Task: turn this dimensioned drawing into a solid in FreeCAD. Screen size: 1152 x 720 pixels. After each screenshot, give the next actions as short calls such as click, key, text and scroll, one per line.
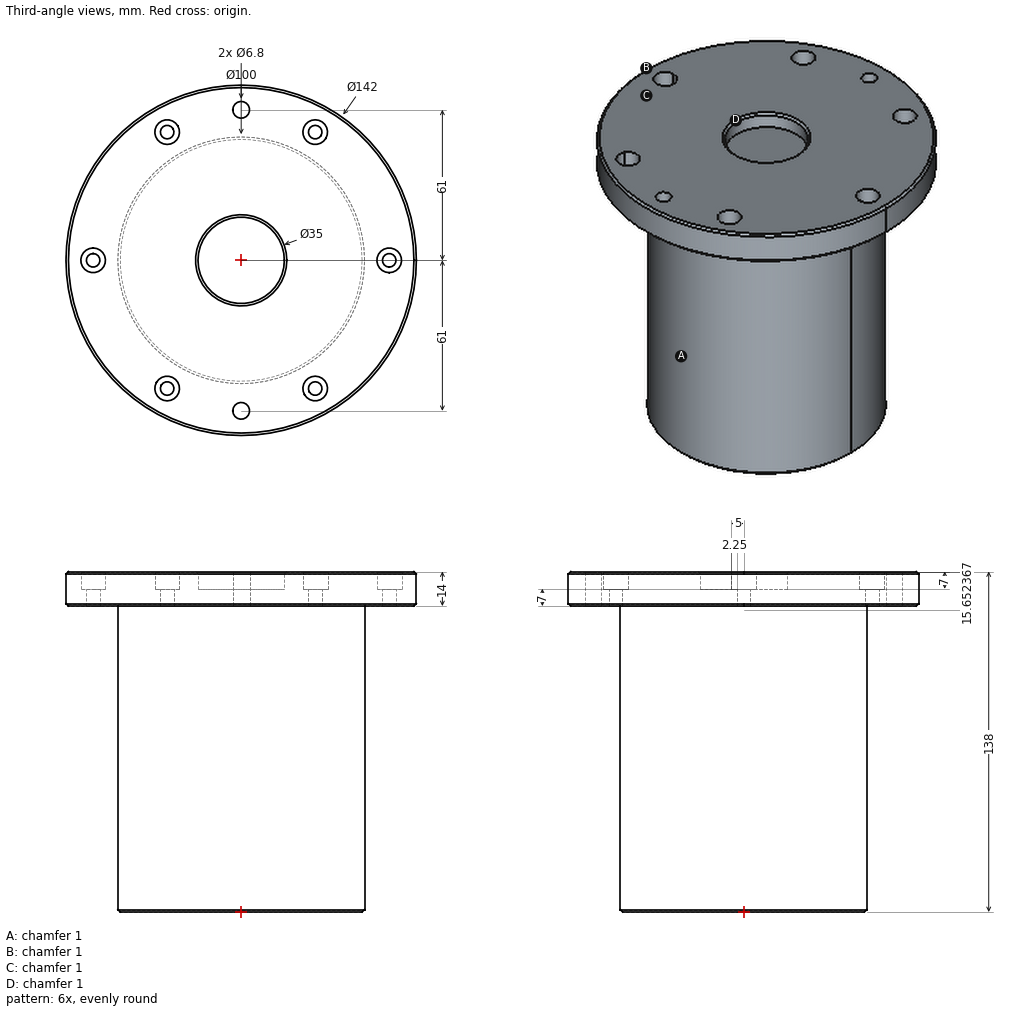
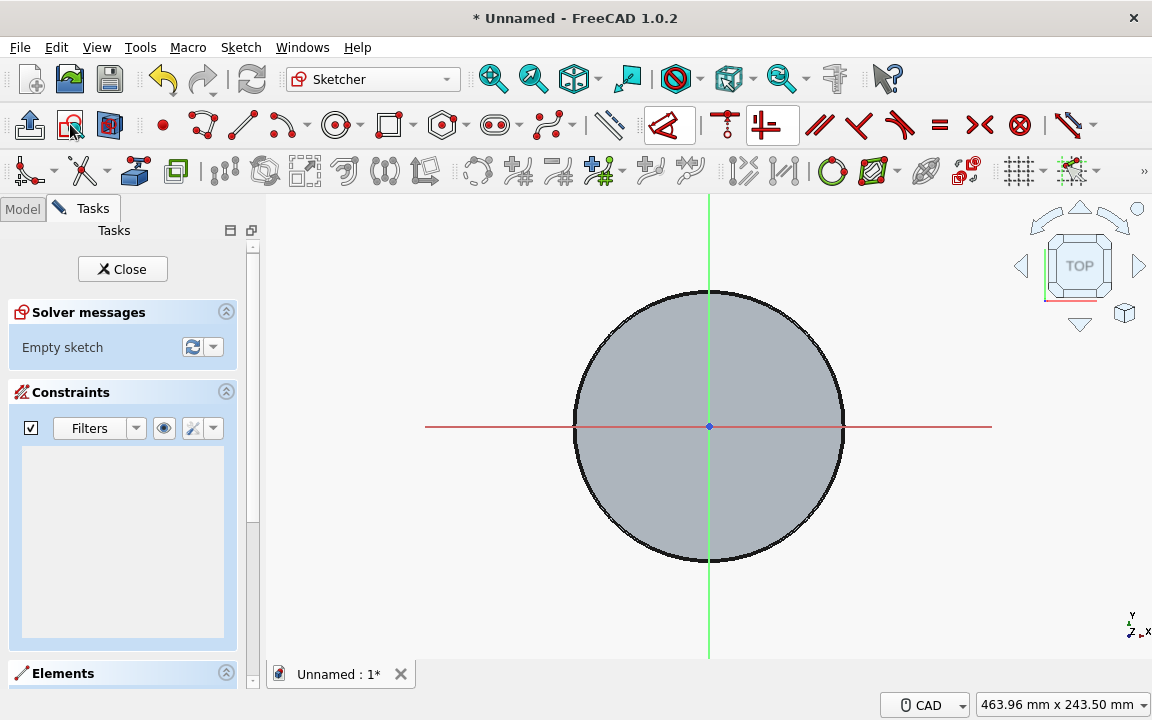
scroll(731, 426, up, 7)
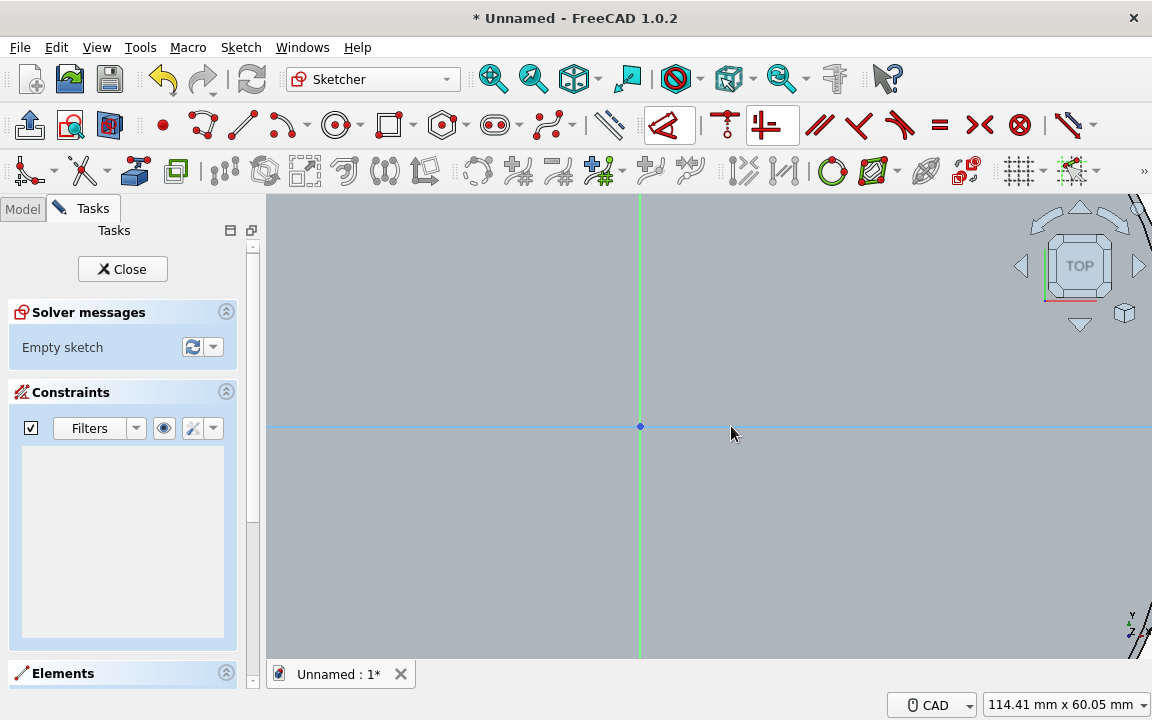
click(336, 126)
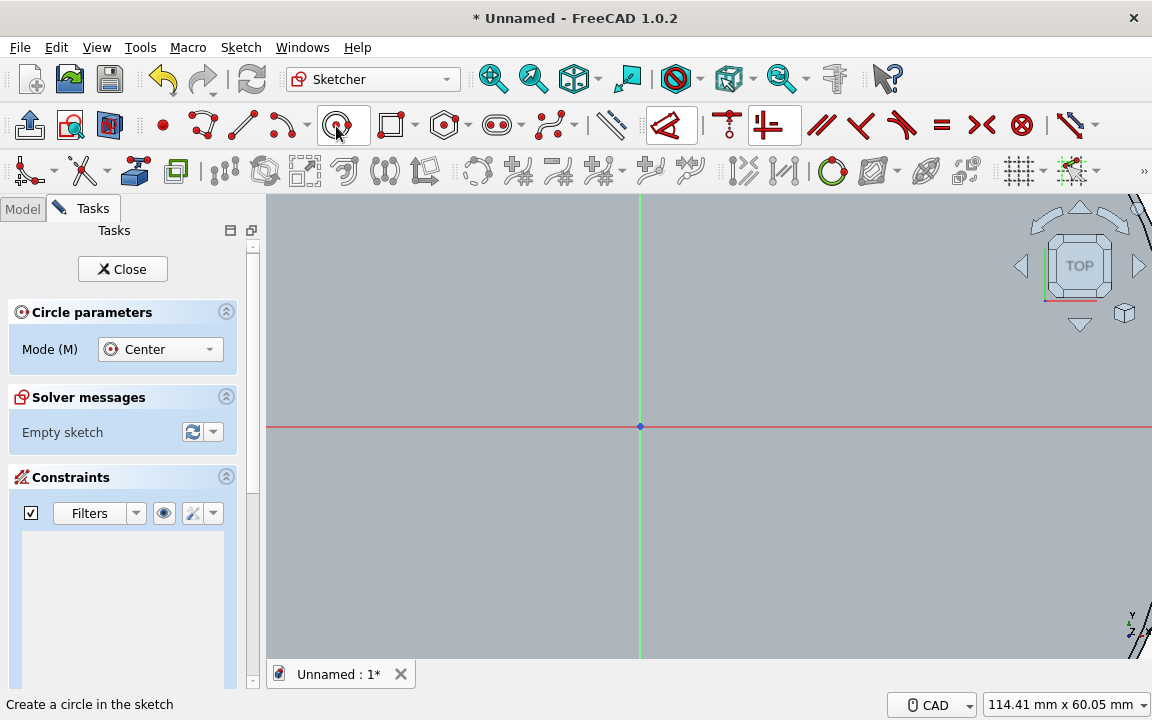
click(640, 426)
click(736, 331)
key(Escape)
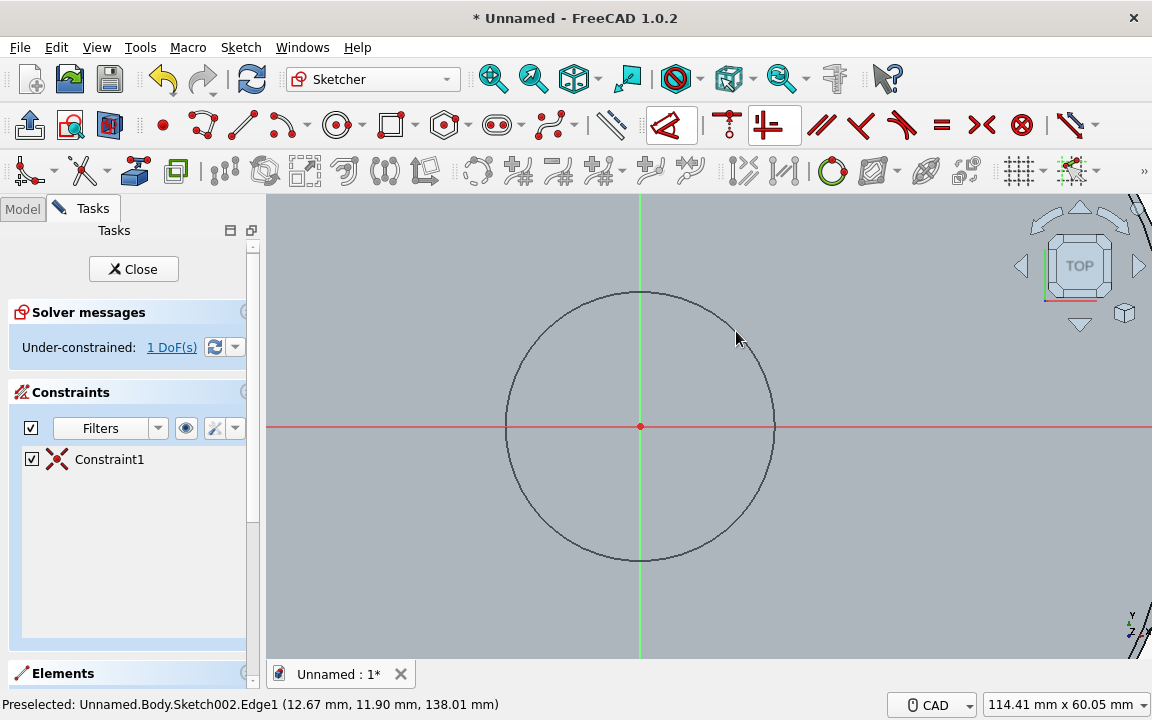
click(735, 331)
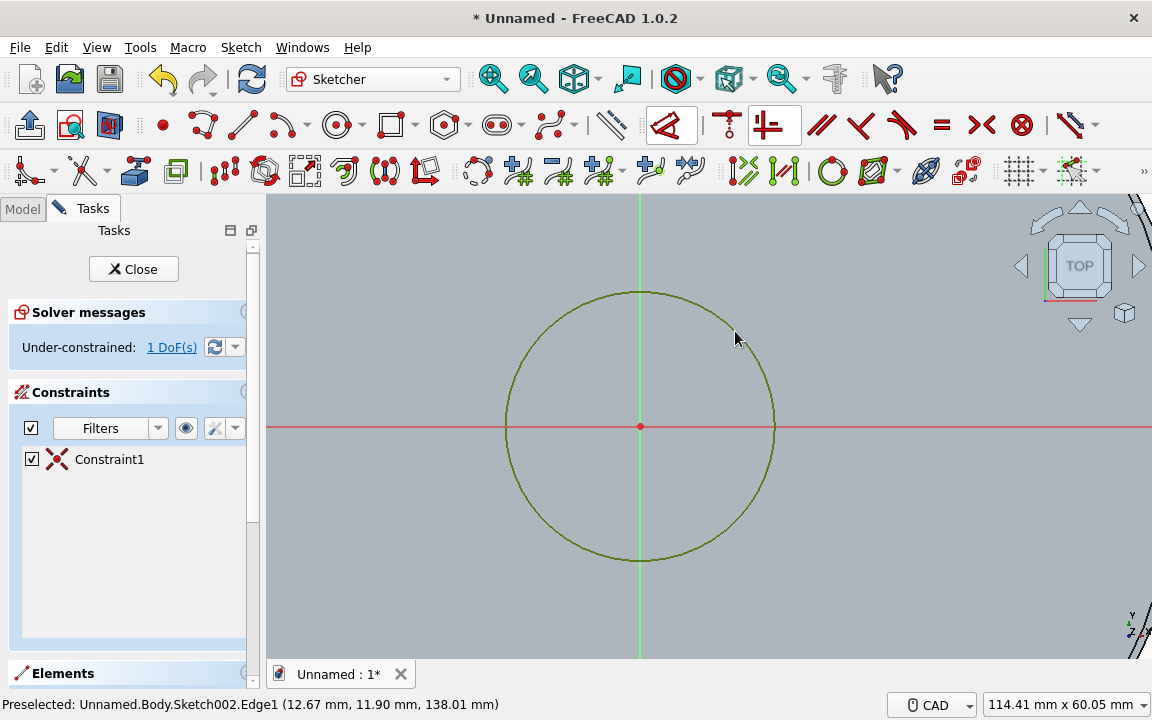
click(692, 126)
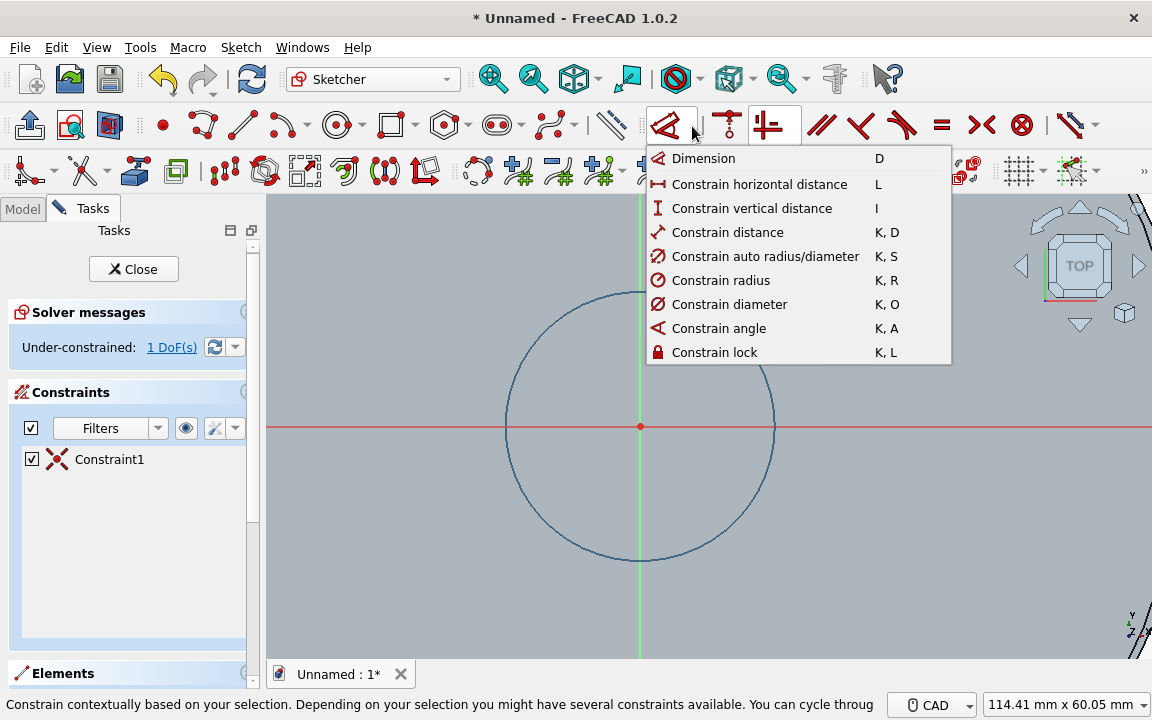
click(799, 304)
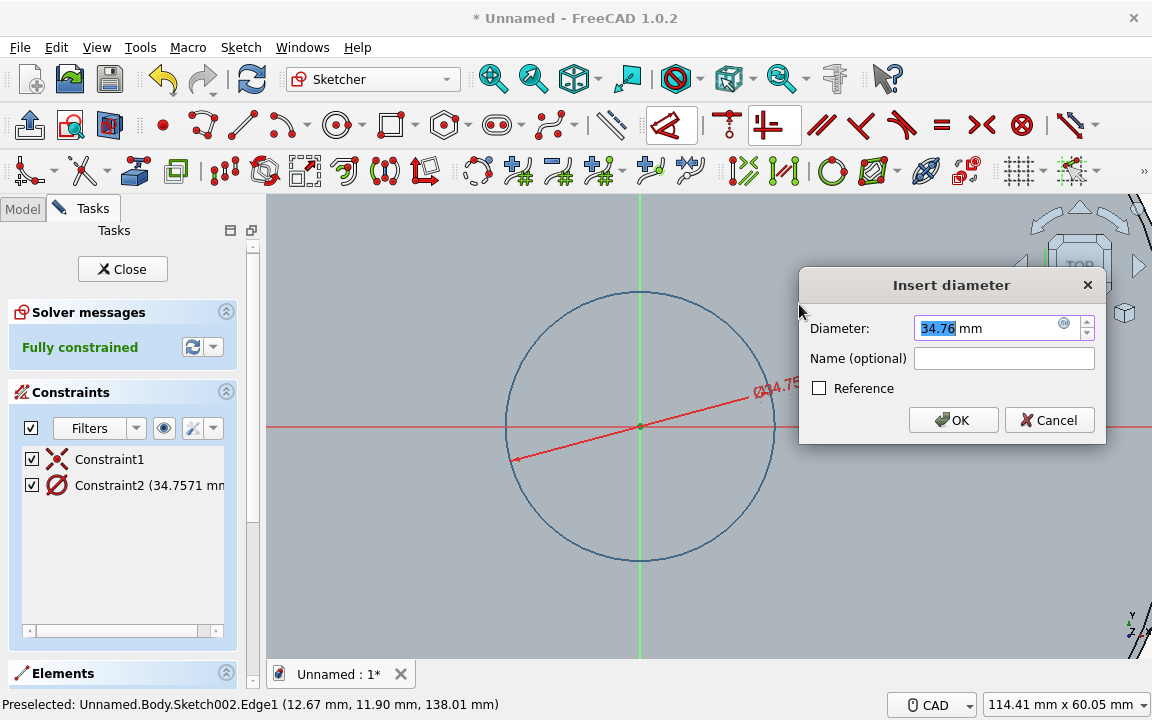
text(35)
key(Return)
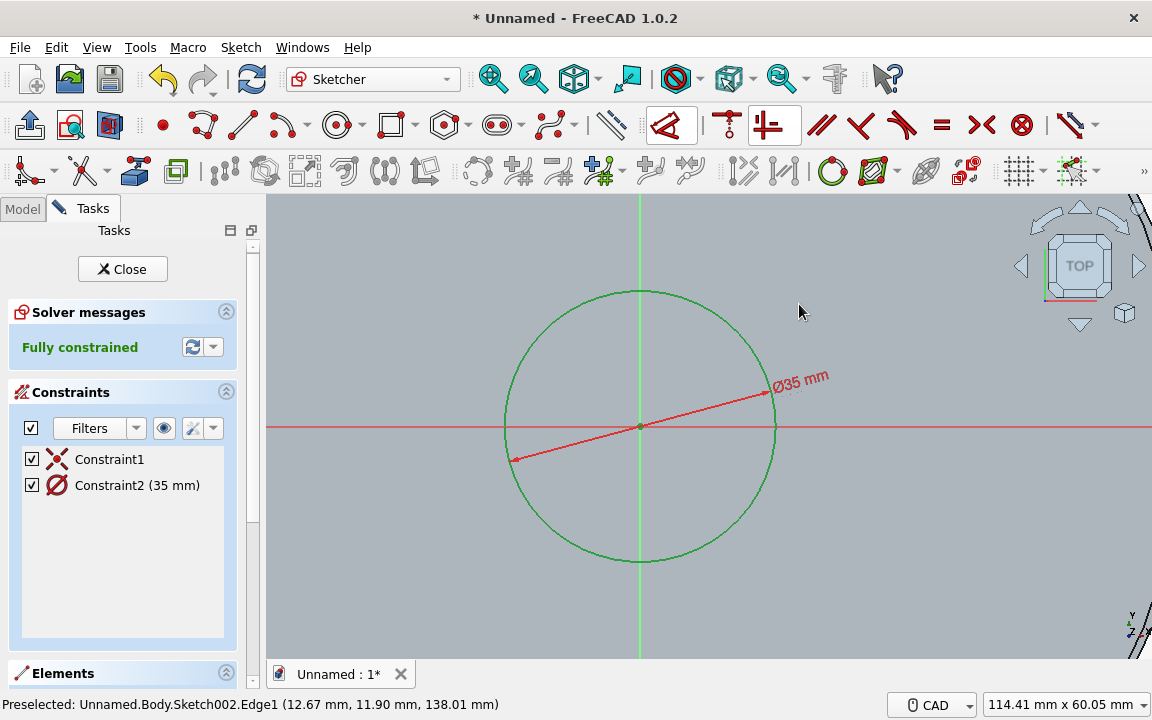
click(123, 269)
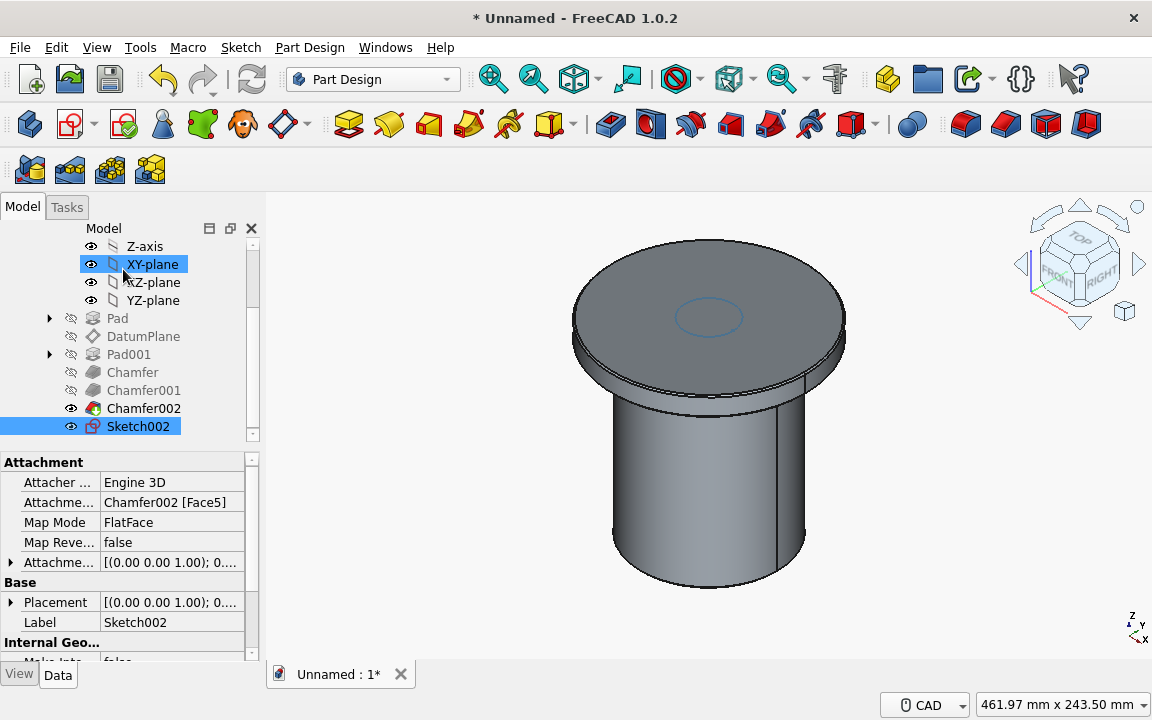
click(612, 124)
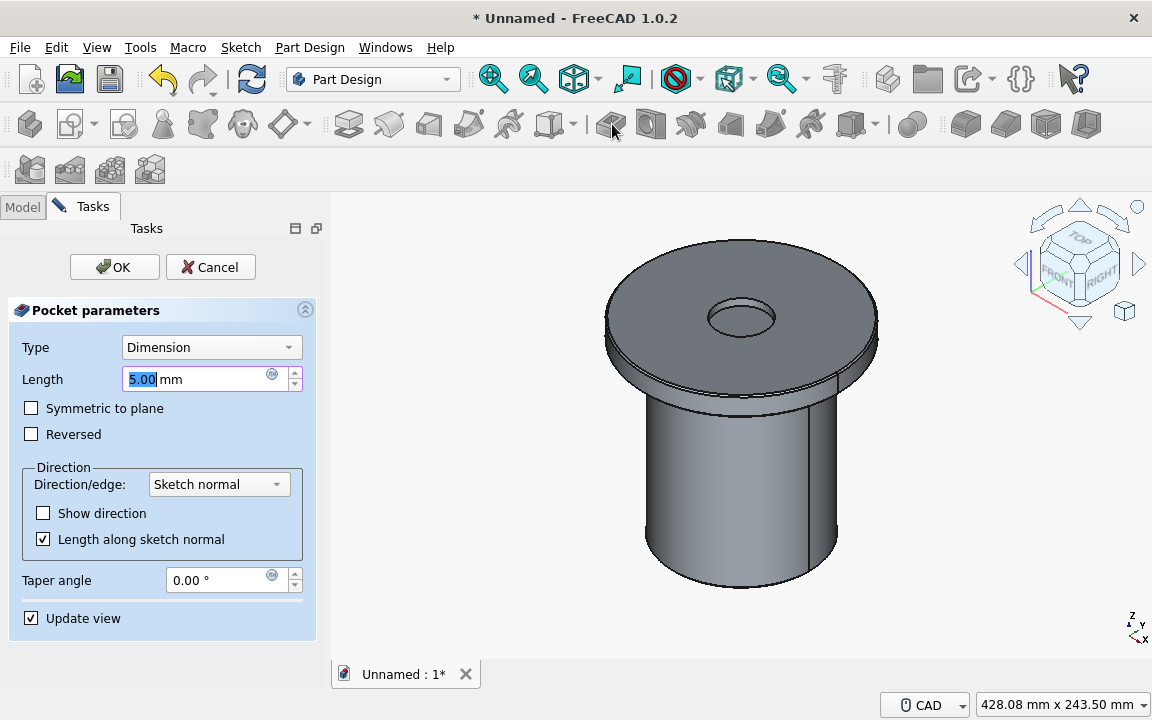
text(7)
key(Tab)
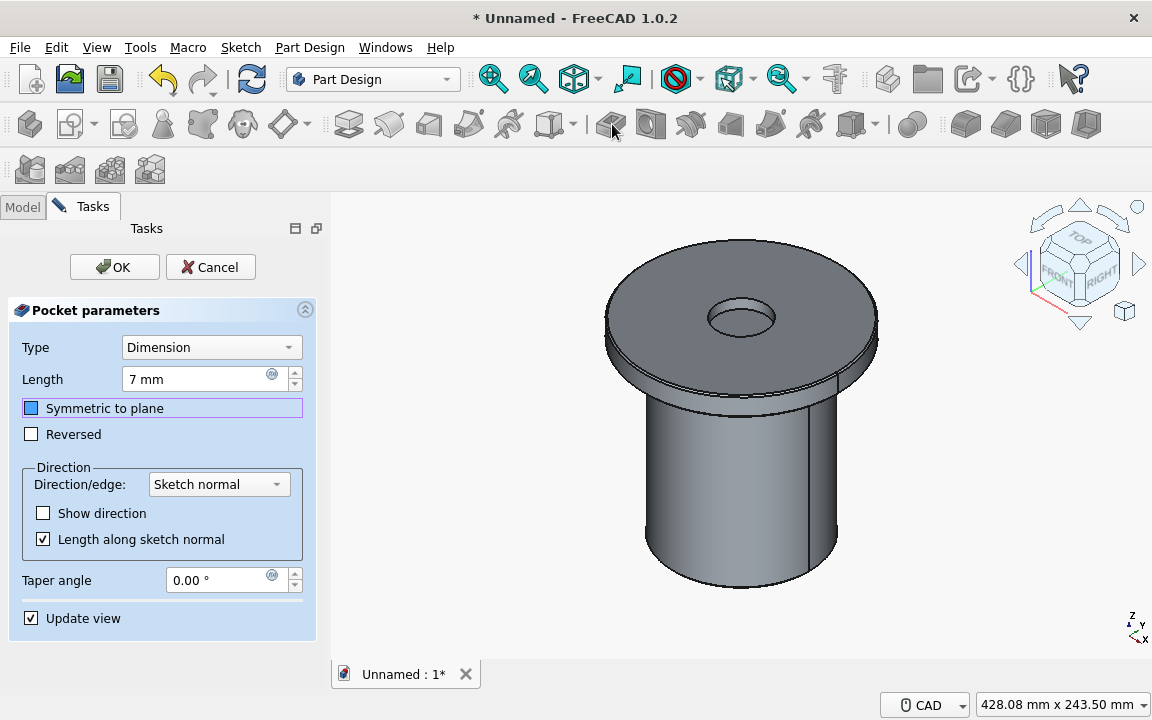
click(115, 267)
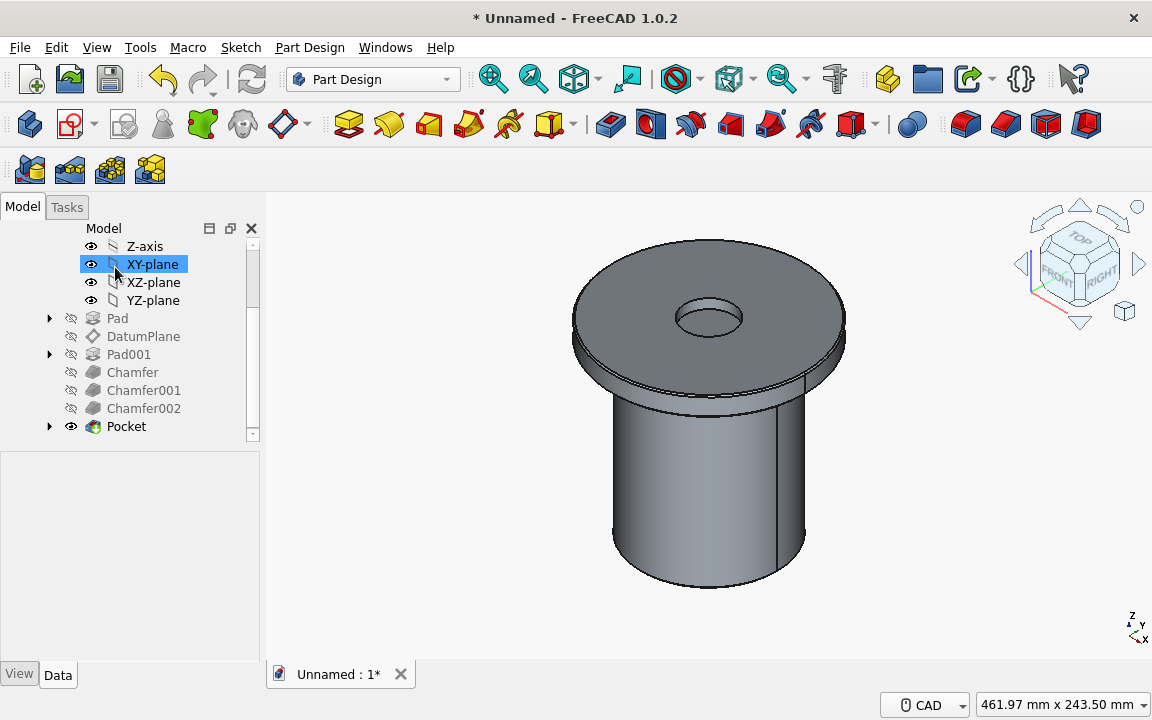
click(685, 303)